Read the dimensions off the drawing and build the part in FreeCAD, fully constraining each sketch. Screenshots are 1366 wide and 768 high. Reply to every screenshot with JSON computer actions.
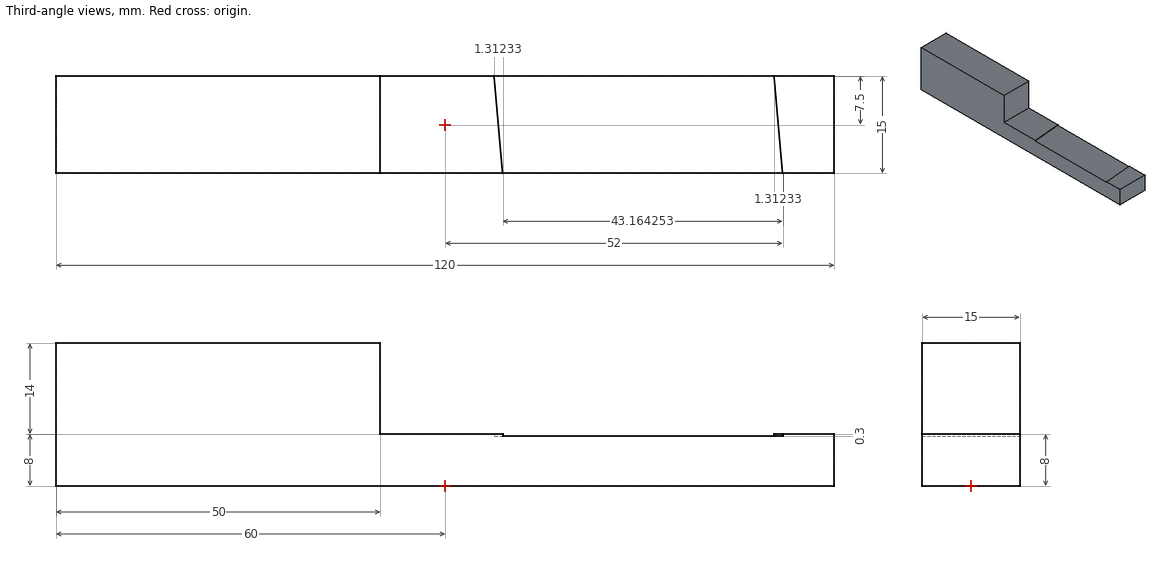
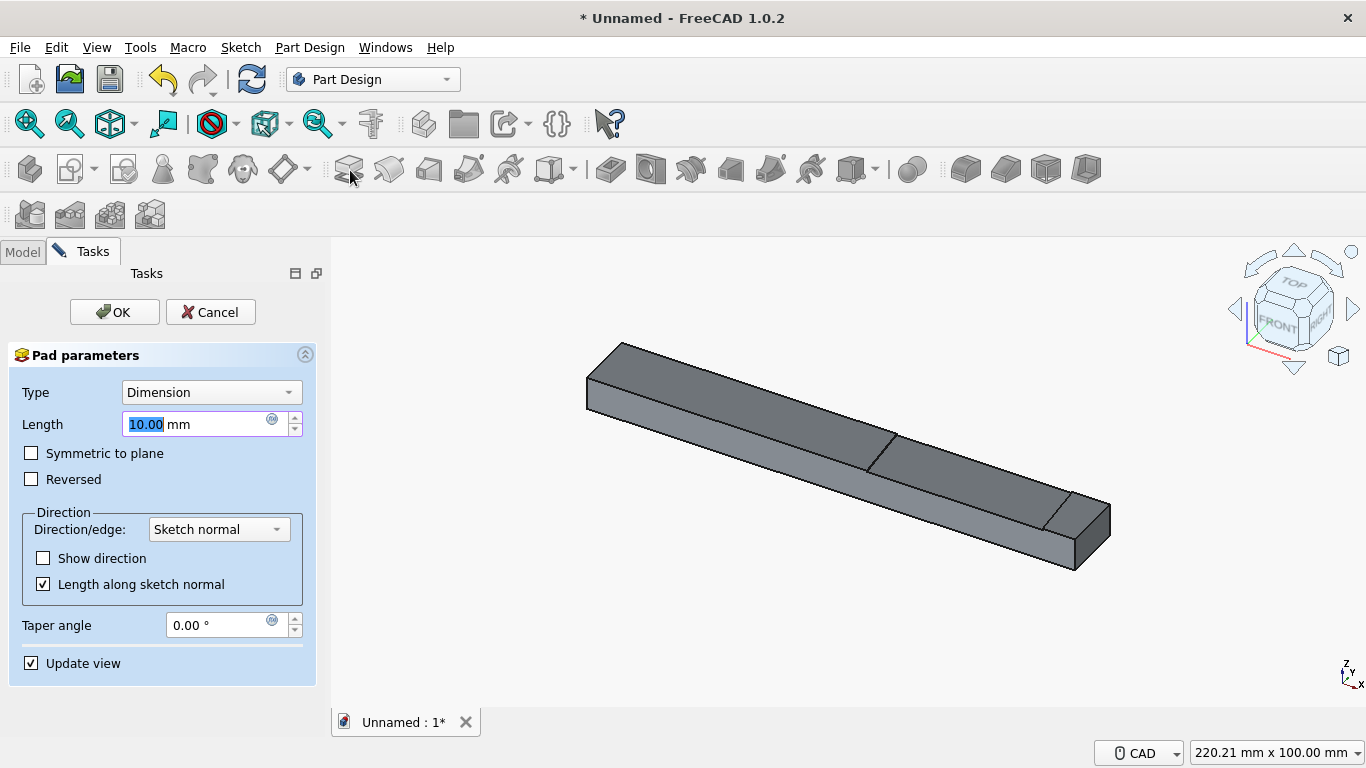
{"action": "type", "text": "15"}
{"action": "key", "text": "Tab"}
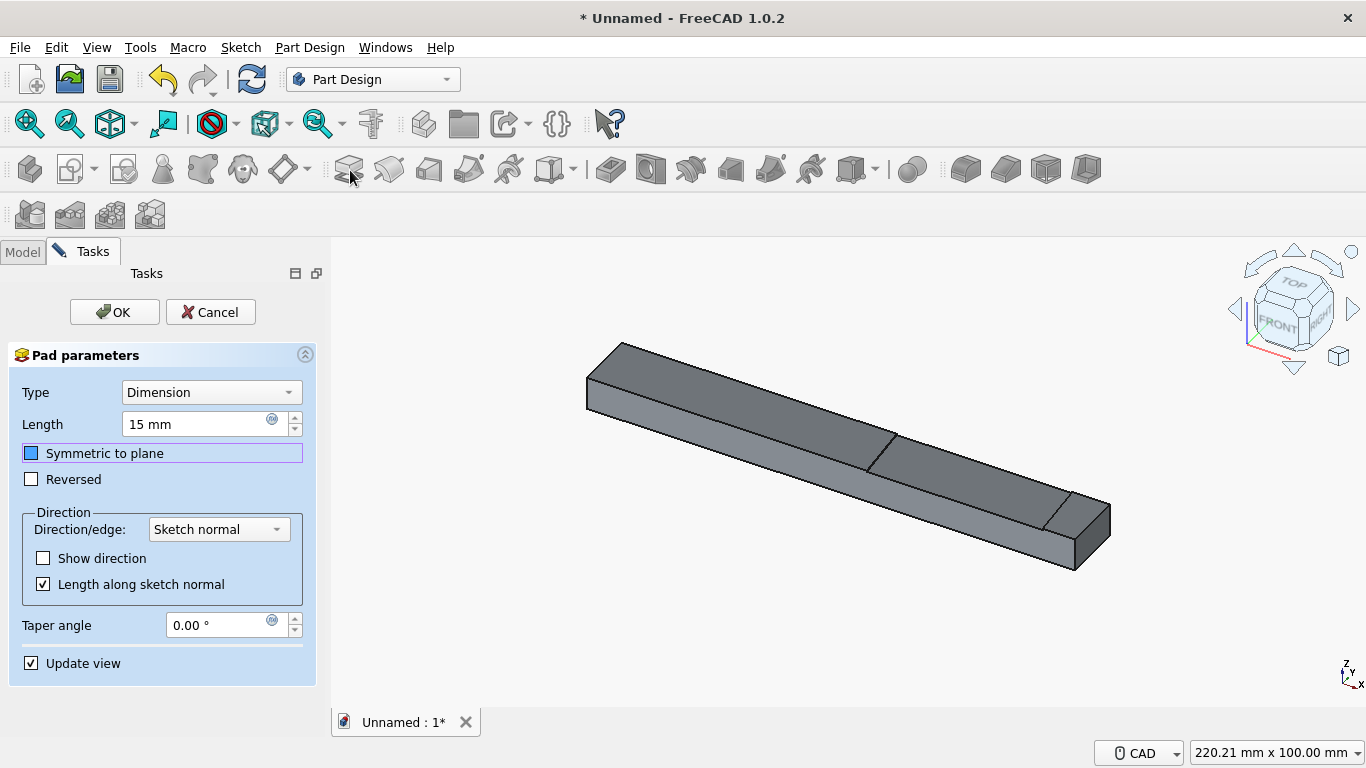
{"action": "left_click", "coordinate": [30, 479]}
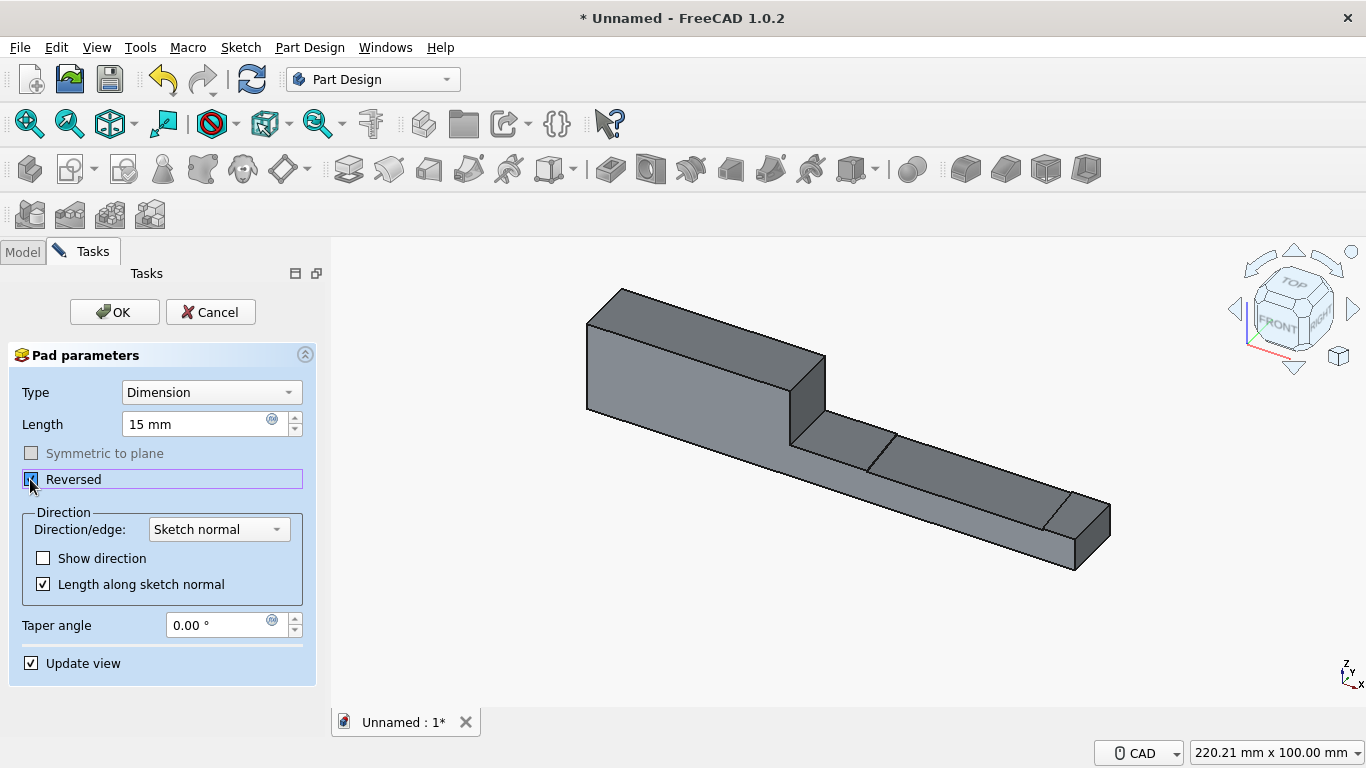
{"action": "left_click", "coordinate": [115, 312]}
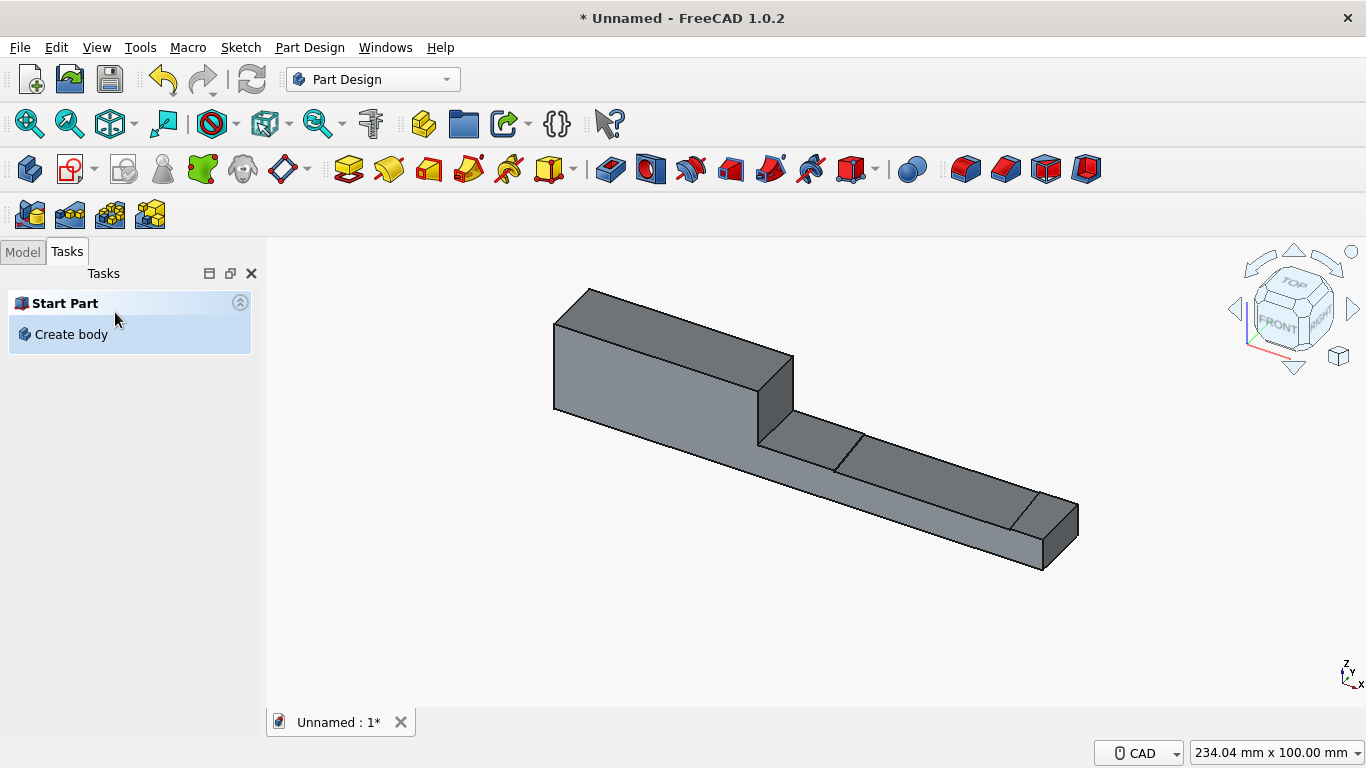
{"action": "key", "text": "0"}